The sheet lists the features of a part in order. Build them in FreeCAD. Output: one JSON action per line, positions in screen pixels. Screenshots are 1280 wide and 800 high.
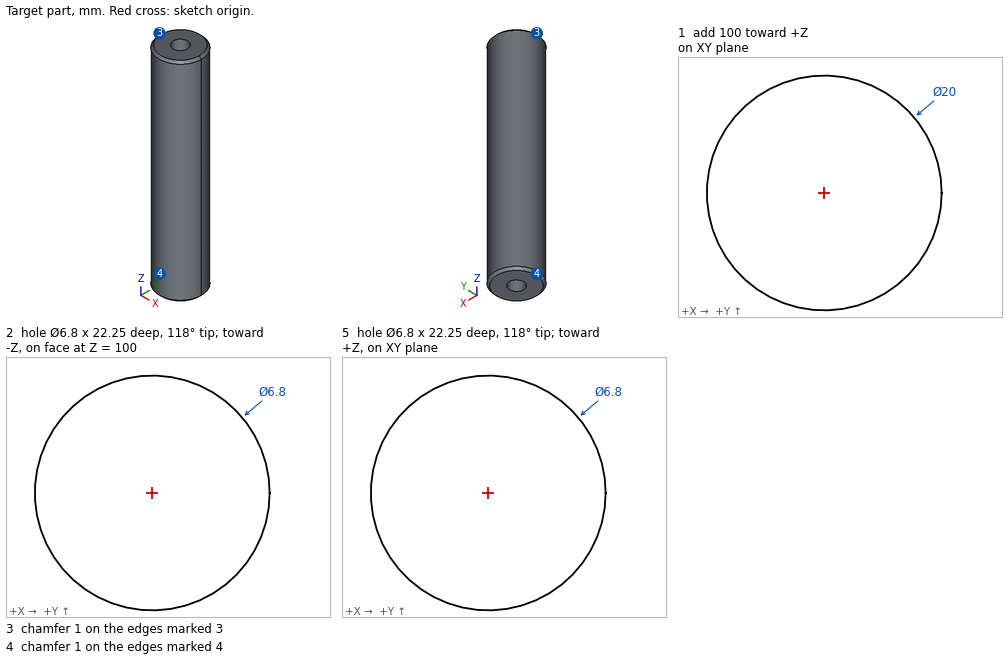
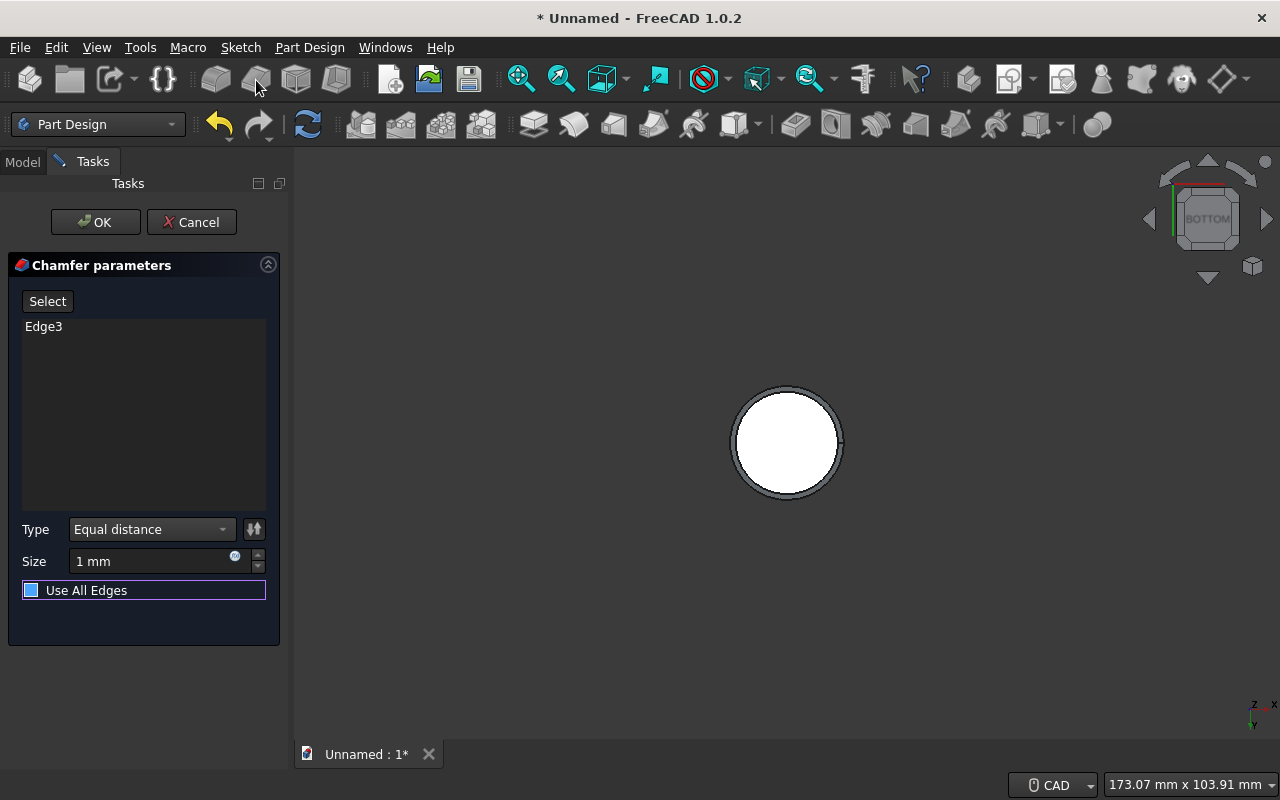
{"action": "left_click", "coordinate": [96, 222]}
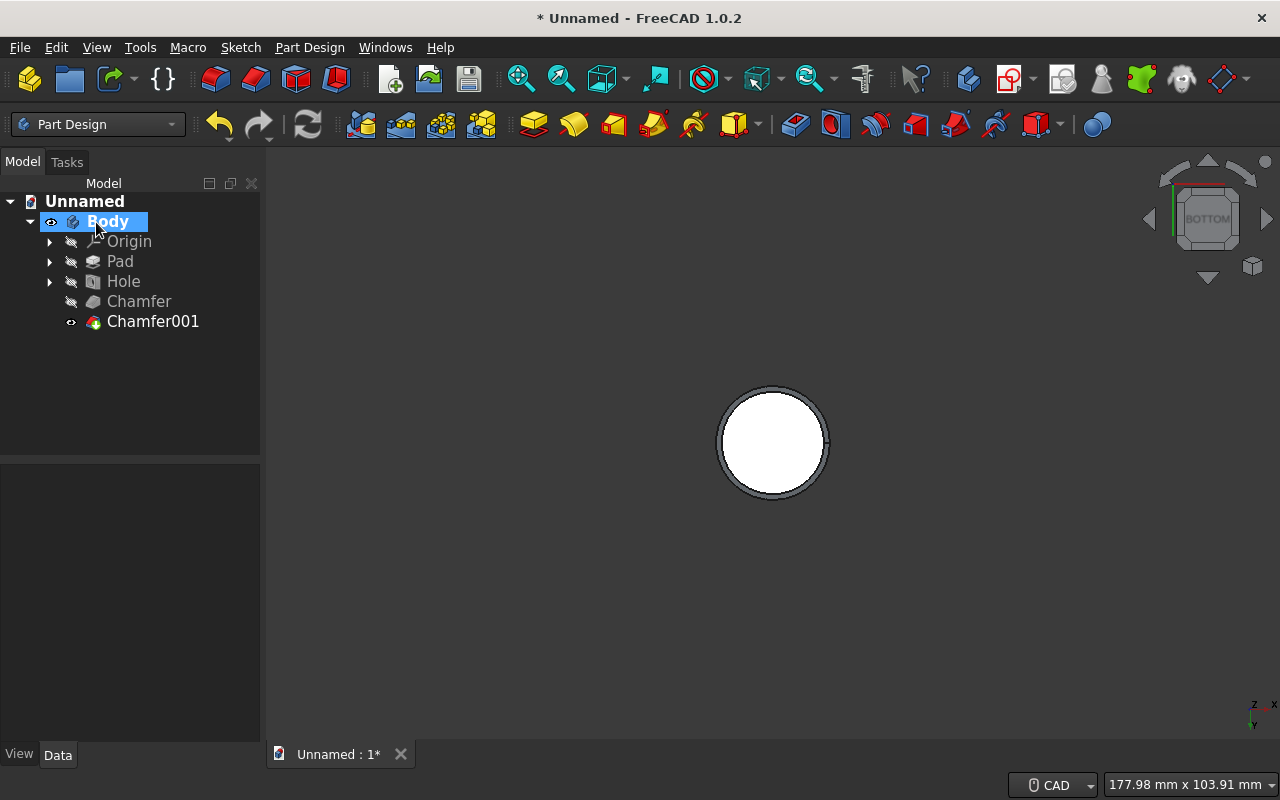
{"action": "left_click", "coordinate": [522, 80]}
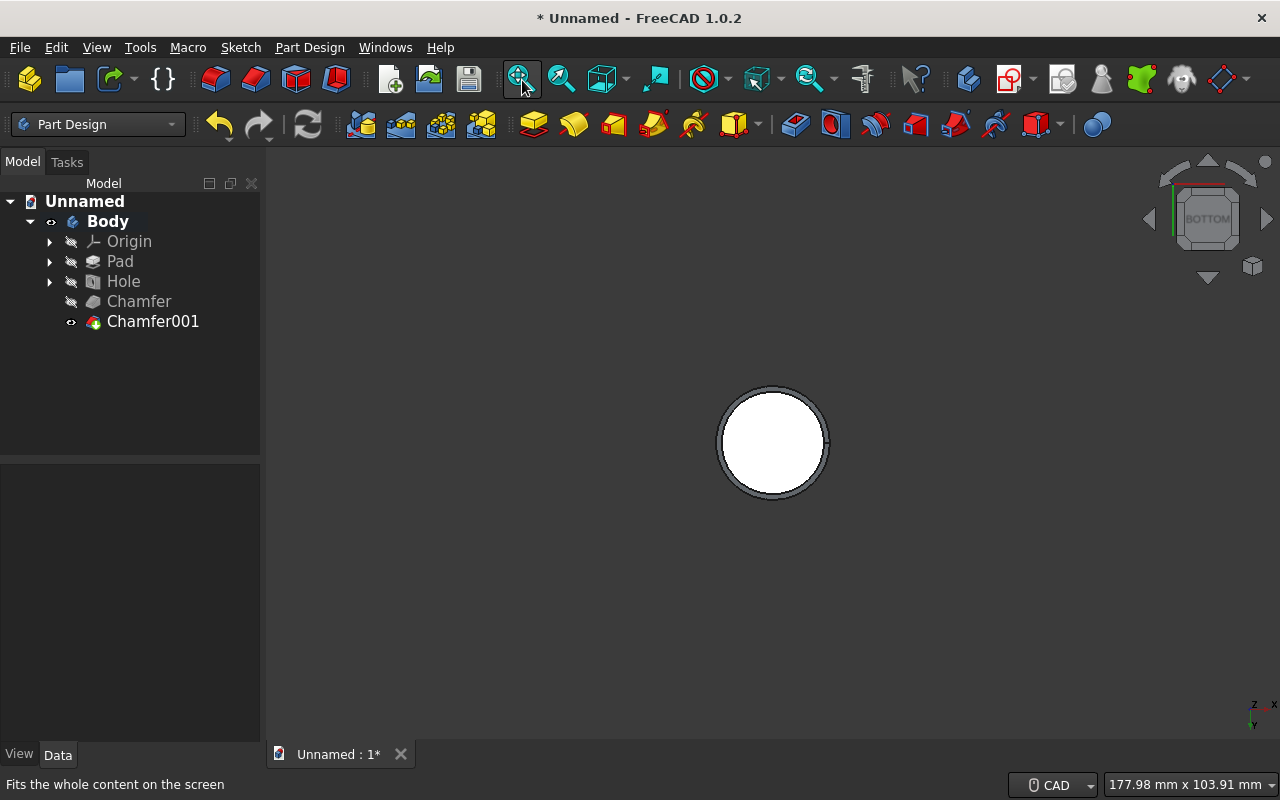
{"action": "left_click", "coordinate": [1010, 80]}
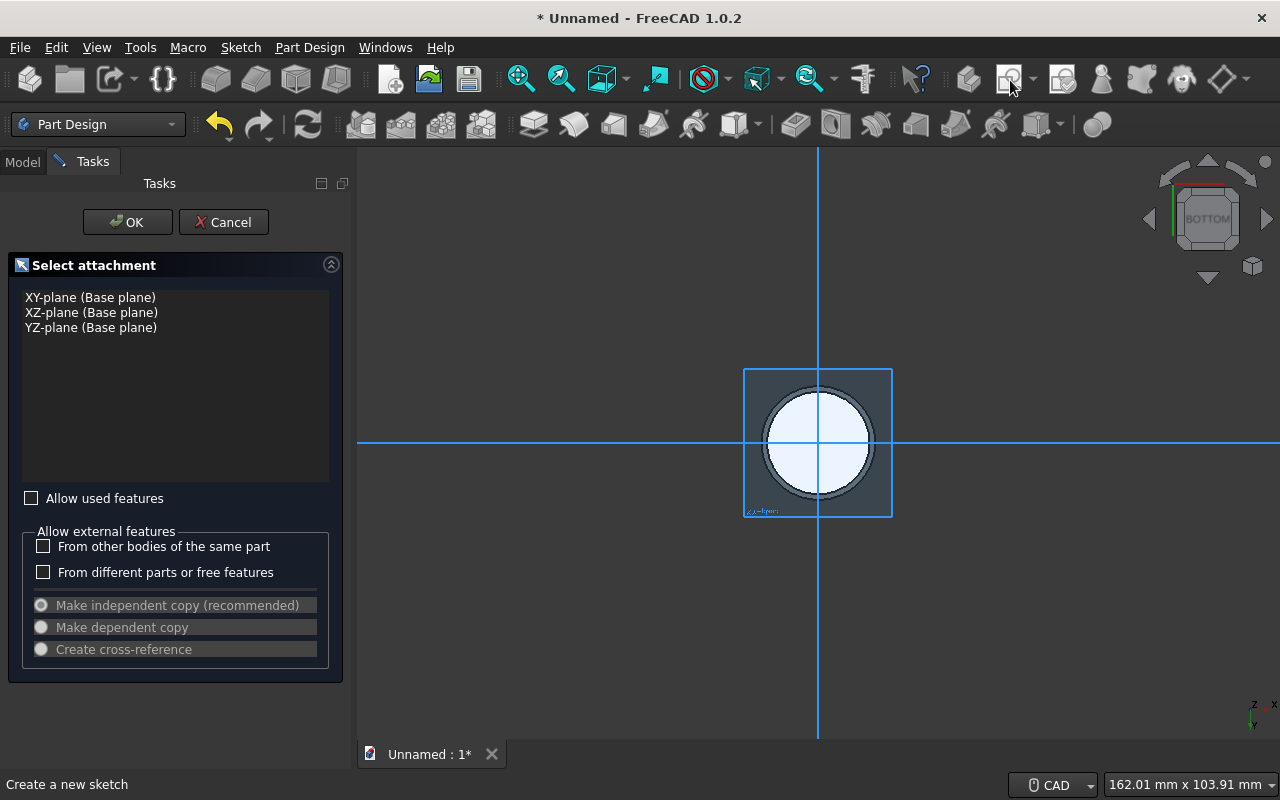
{"action": "left_click", "coordinate": [82, 298]}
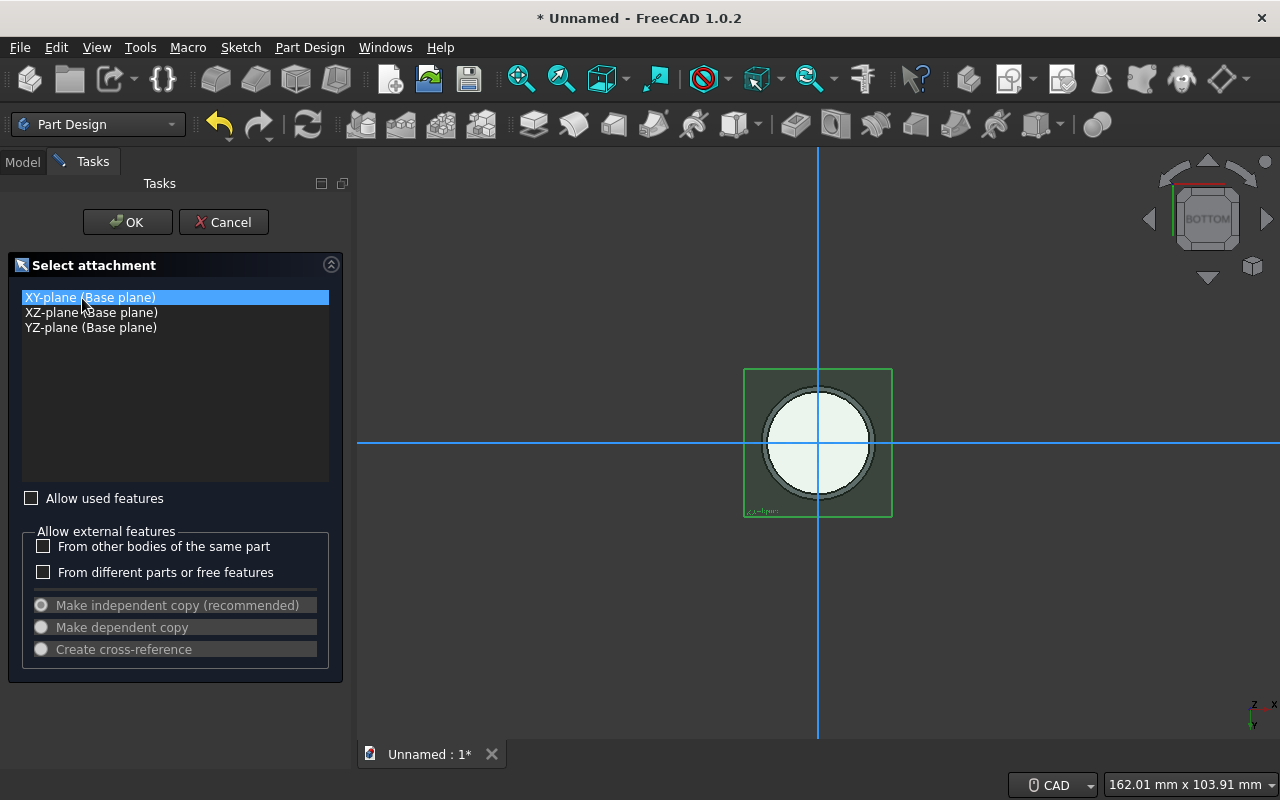
{"action": "left_click", "coordinate": [128, 222]}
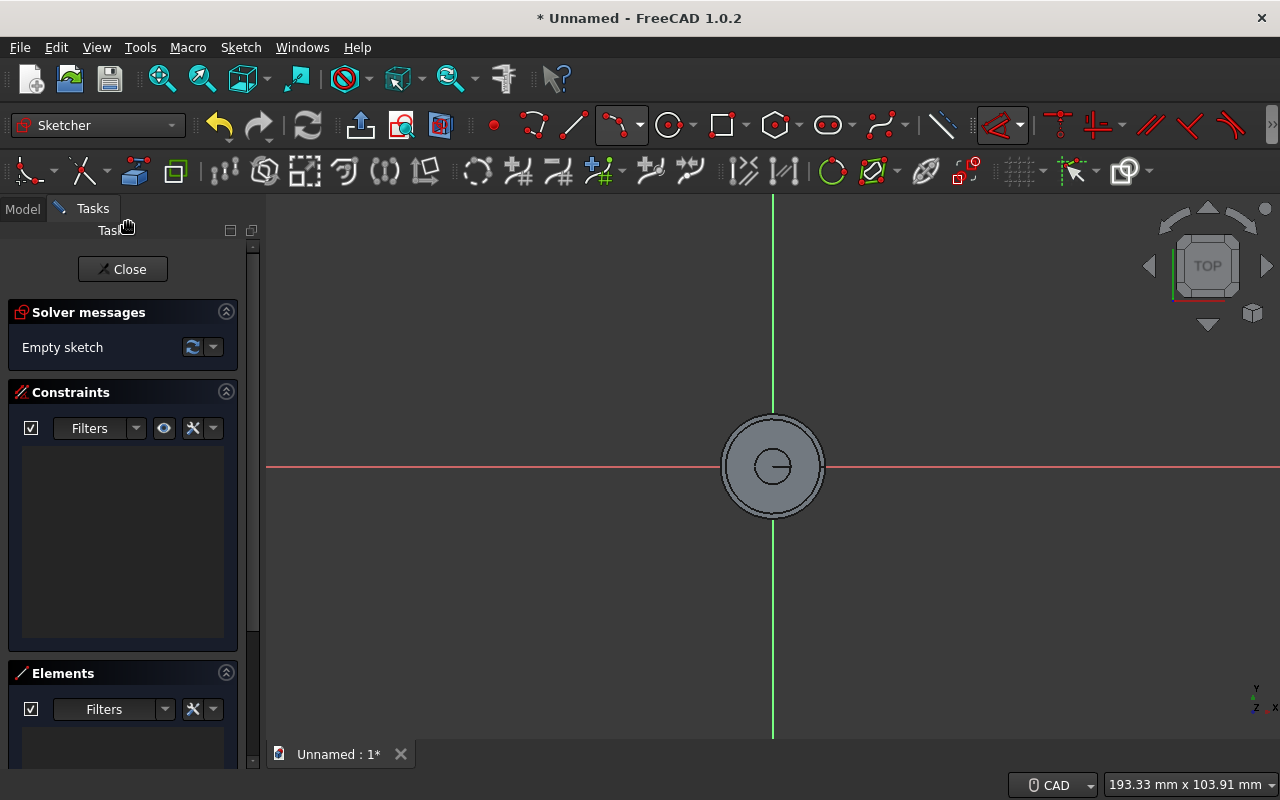
{"action": "key", "text": "q s"}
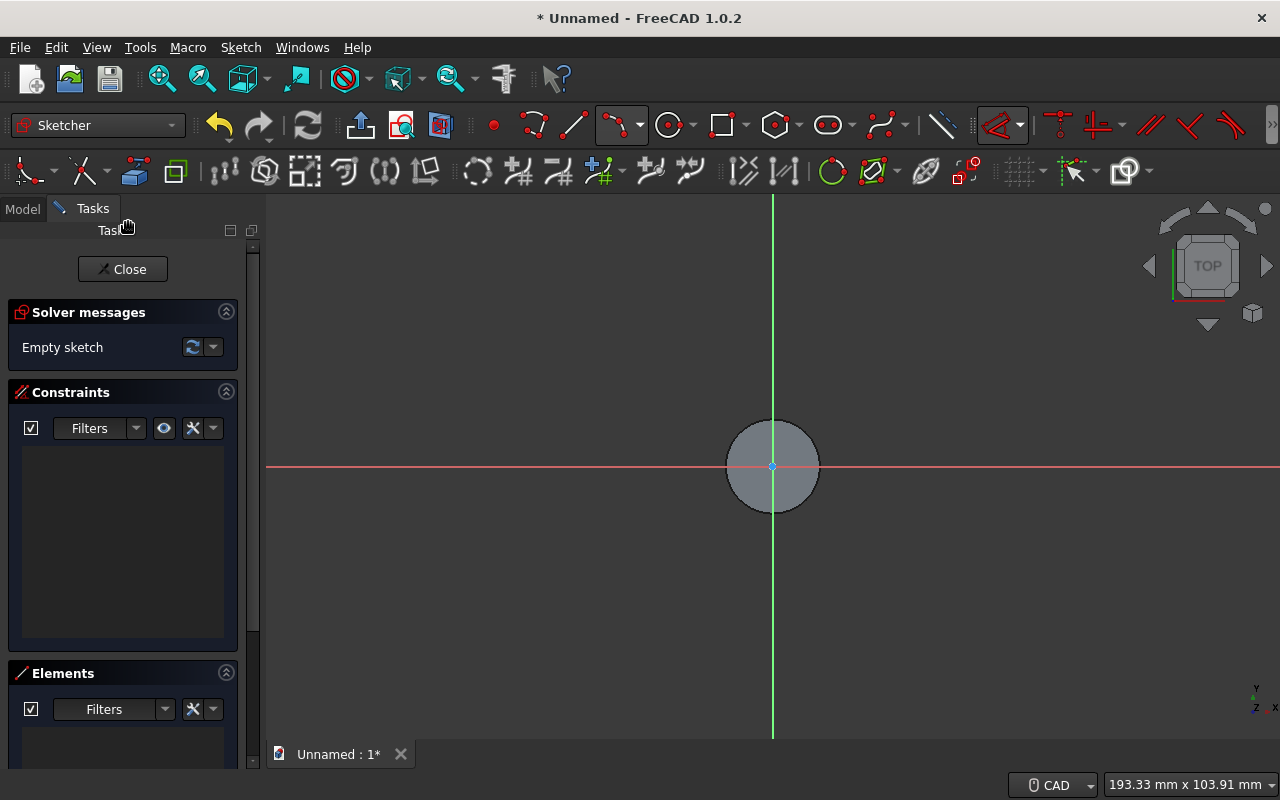
{"action": "scroll", "coordinate": [781, 466], "scroll_direction": "up", "scroll_amount": 11}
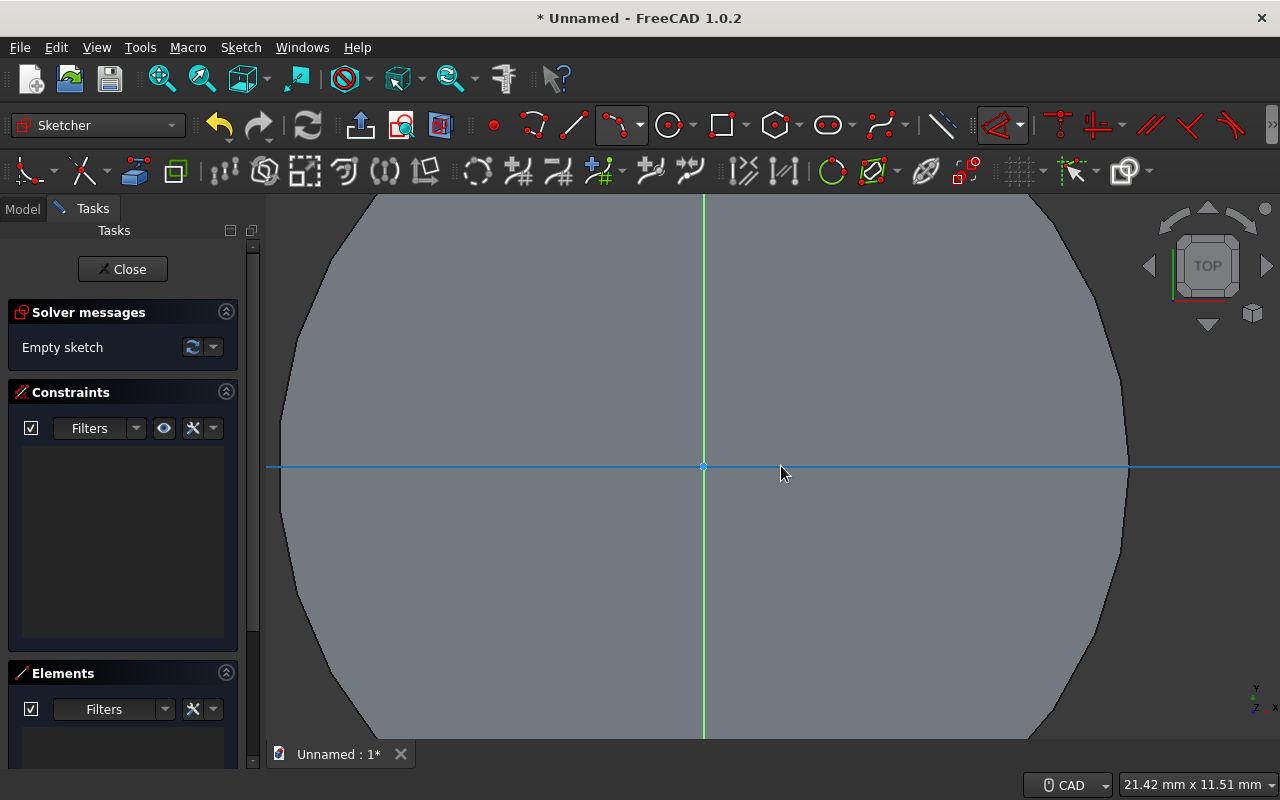
{"action": "key", "text": "g c"}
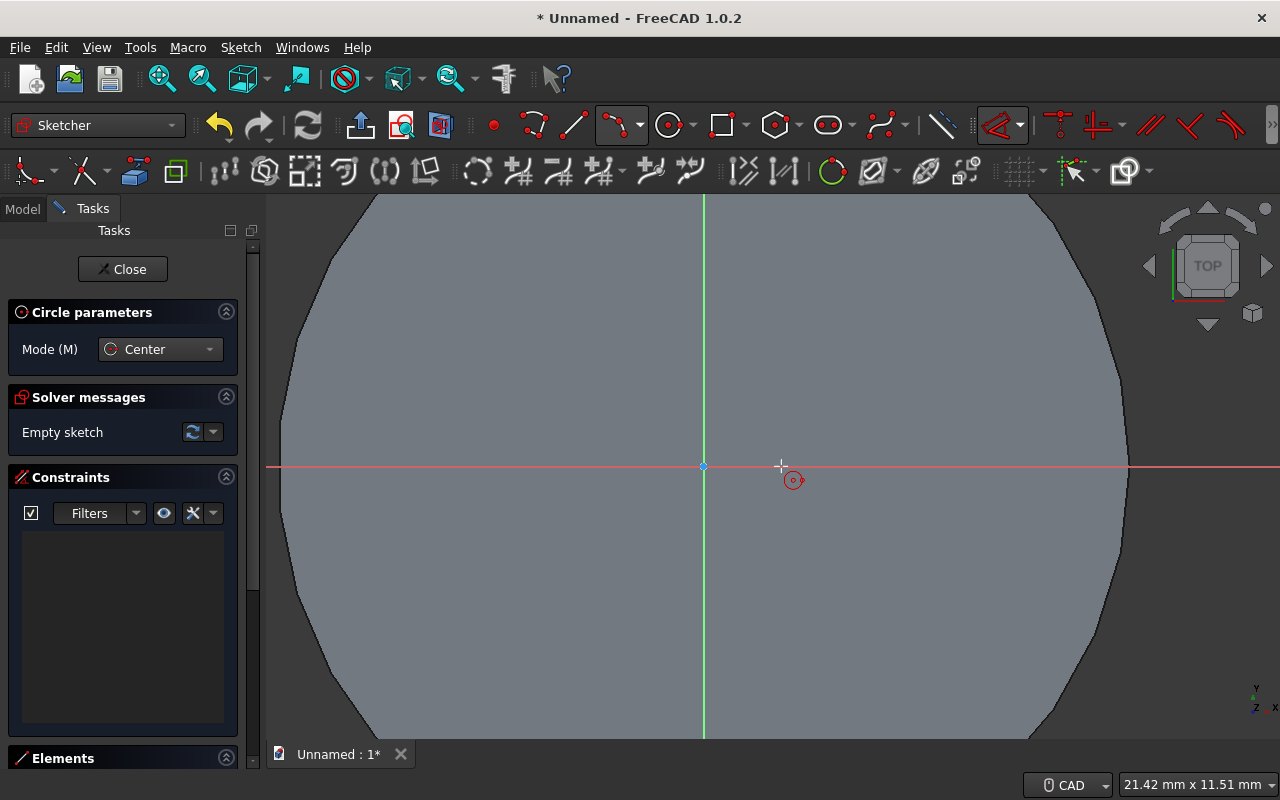
{"action": "left_click", "coordinate": [704, 466]}
{"action": "mouse_move", "coordinate": [817, 353]}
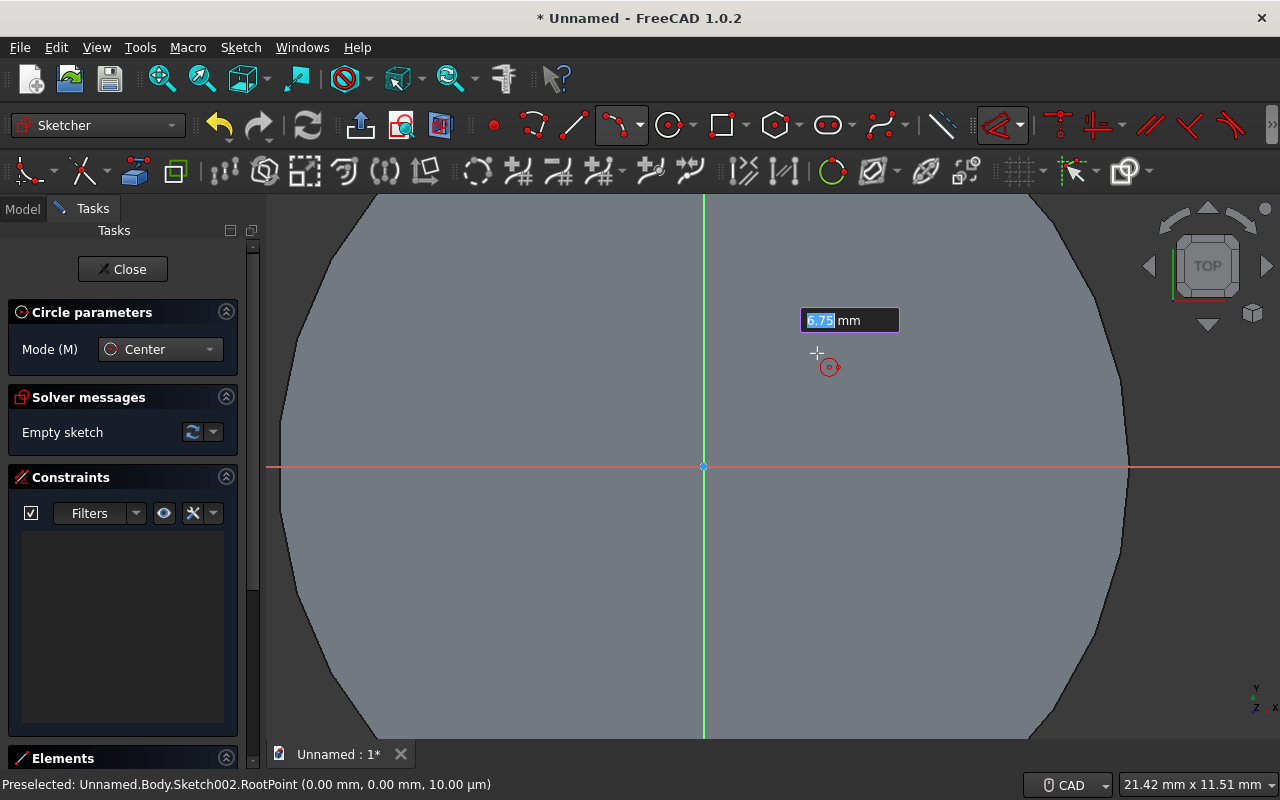
{"action": "type", "text": "6.8"}
{"action": "key", "text": "Return"}
{"action": "key", "text": "Escape"}